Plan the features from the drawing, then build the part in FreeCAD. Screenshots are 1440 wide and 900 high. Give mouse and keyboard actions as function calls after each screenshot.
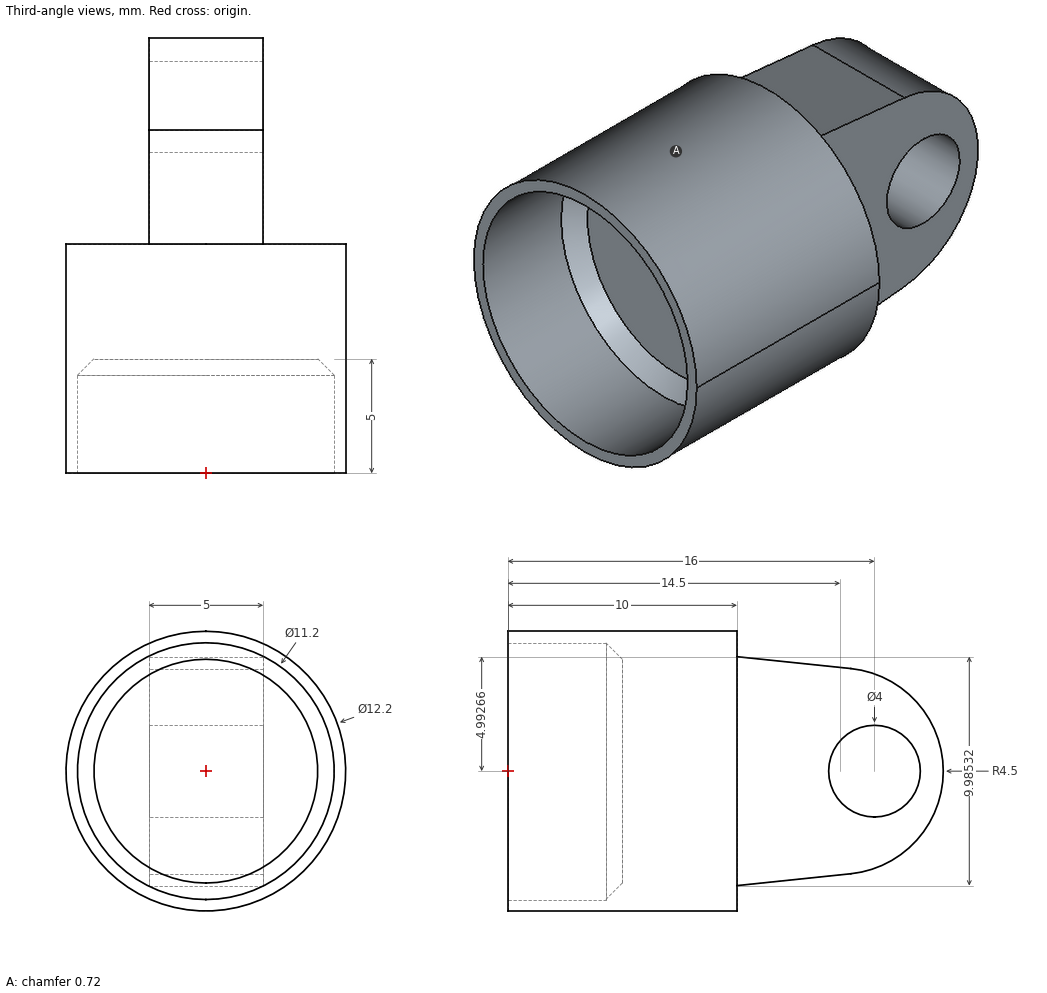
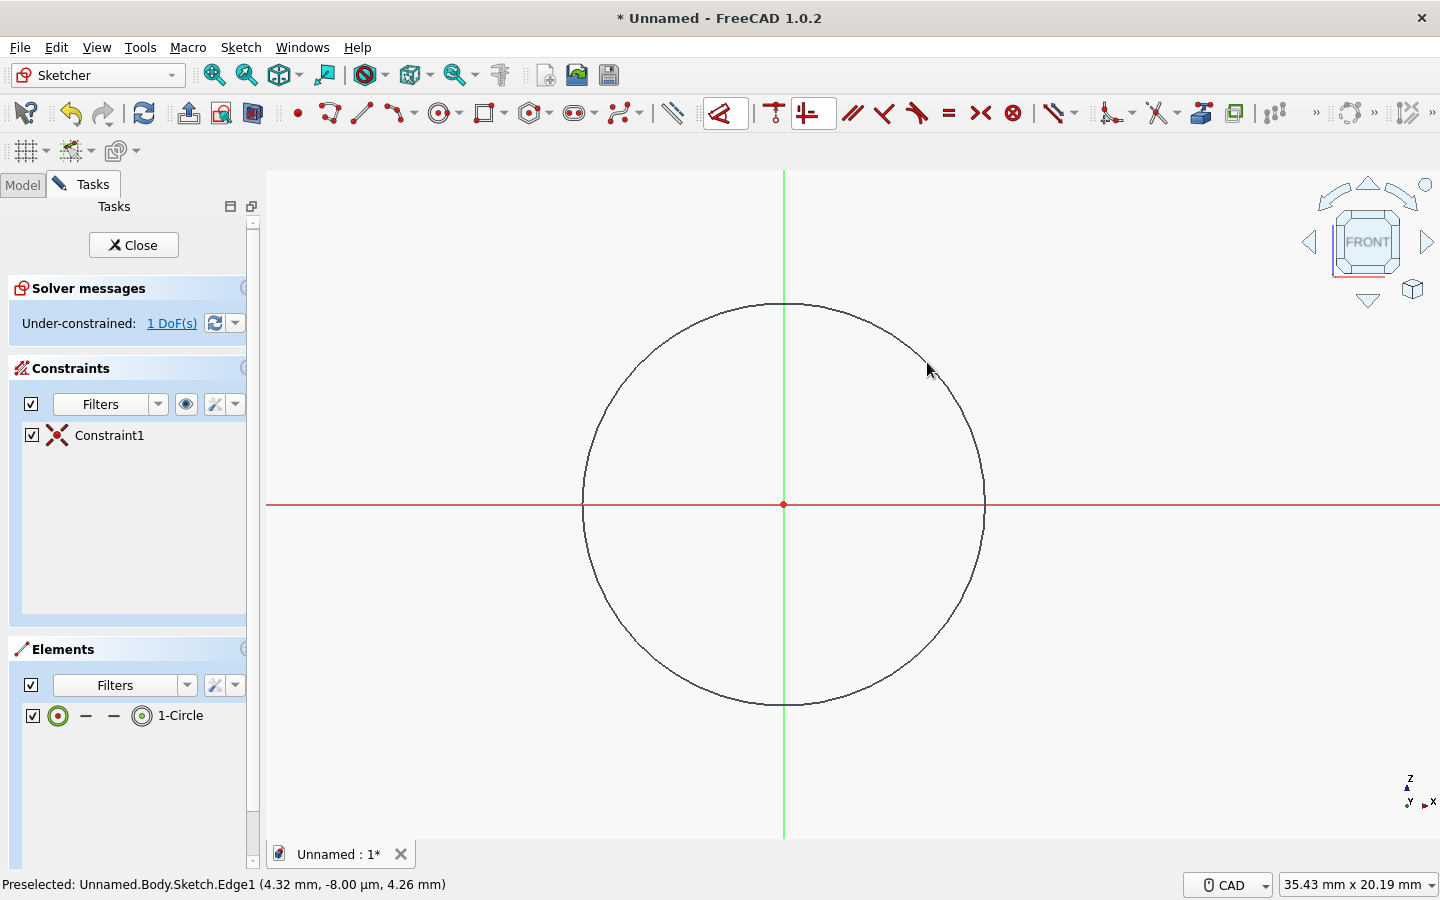
key(d)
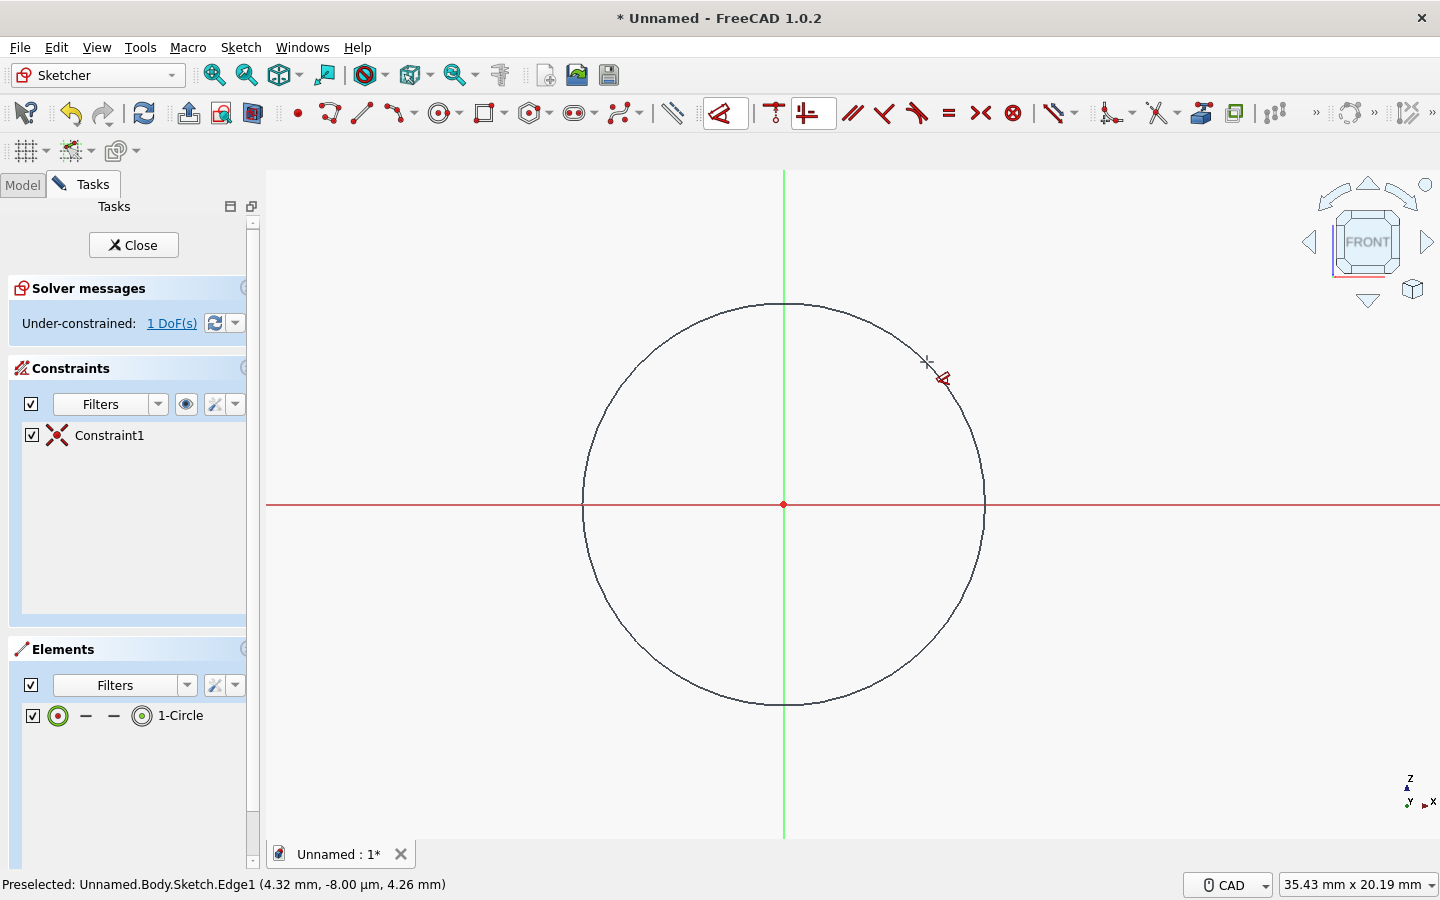
click(926, 362)
click(949, 339)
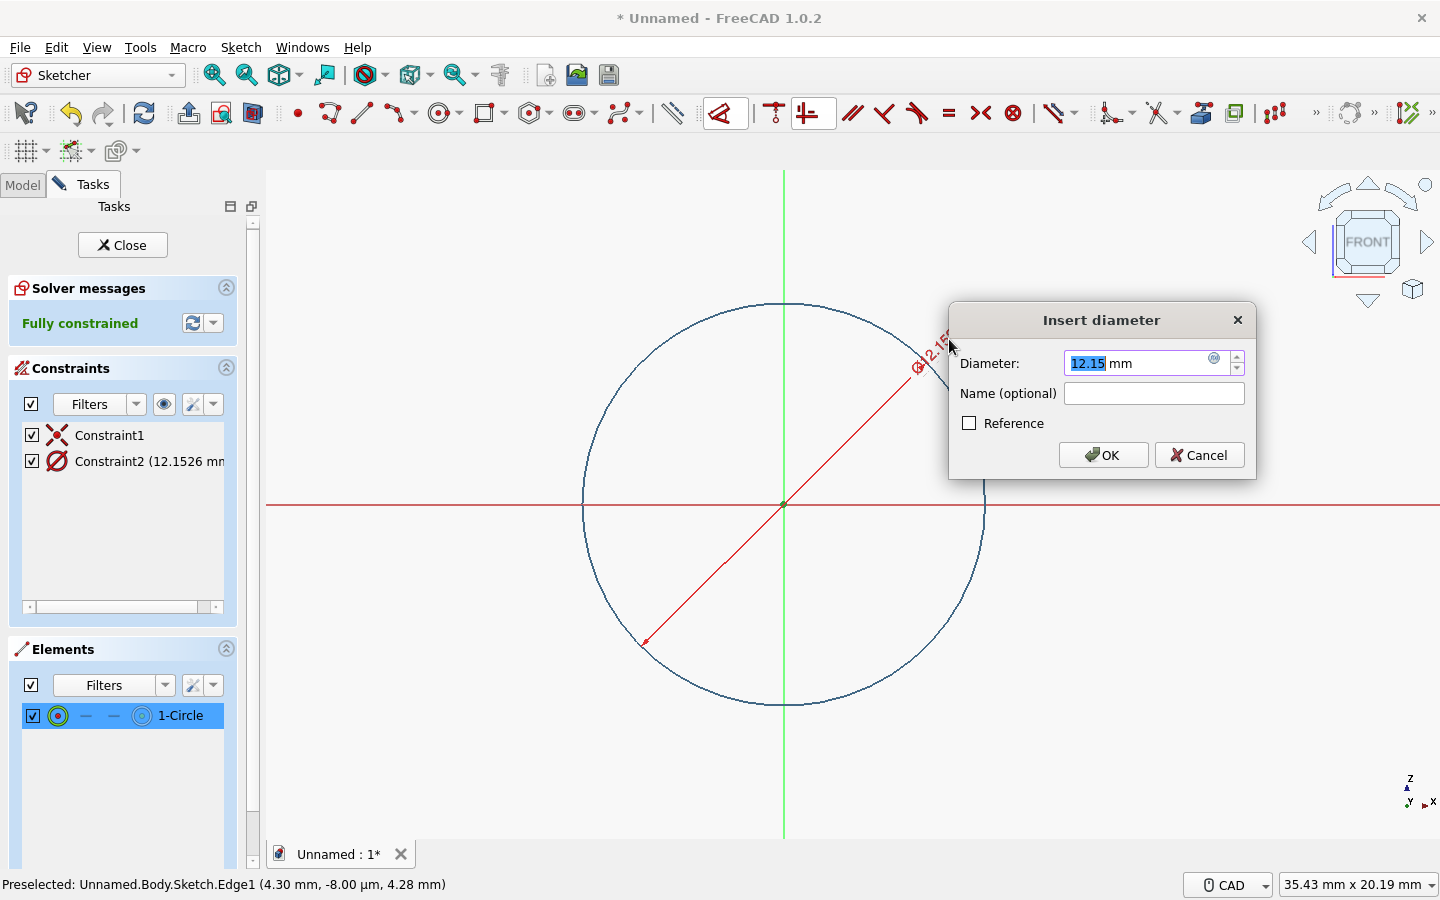
text(12.2)
key(Return)
key(Escape)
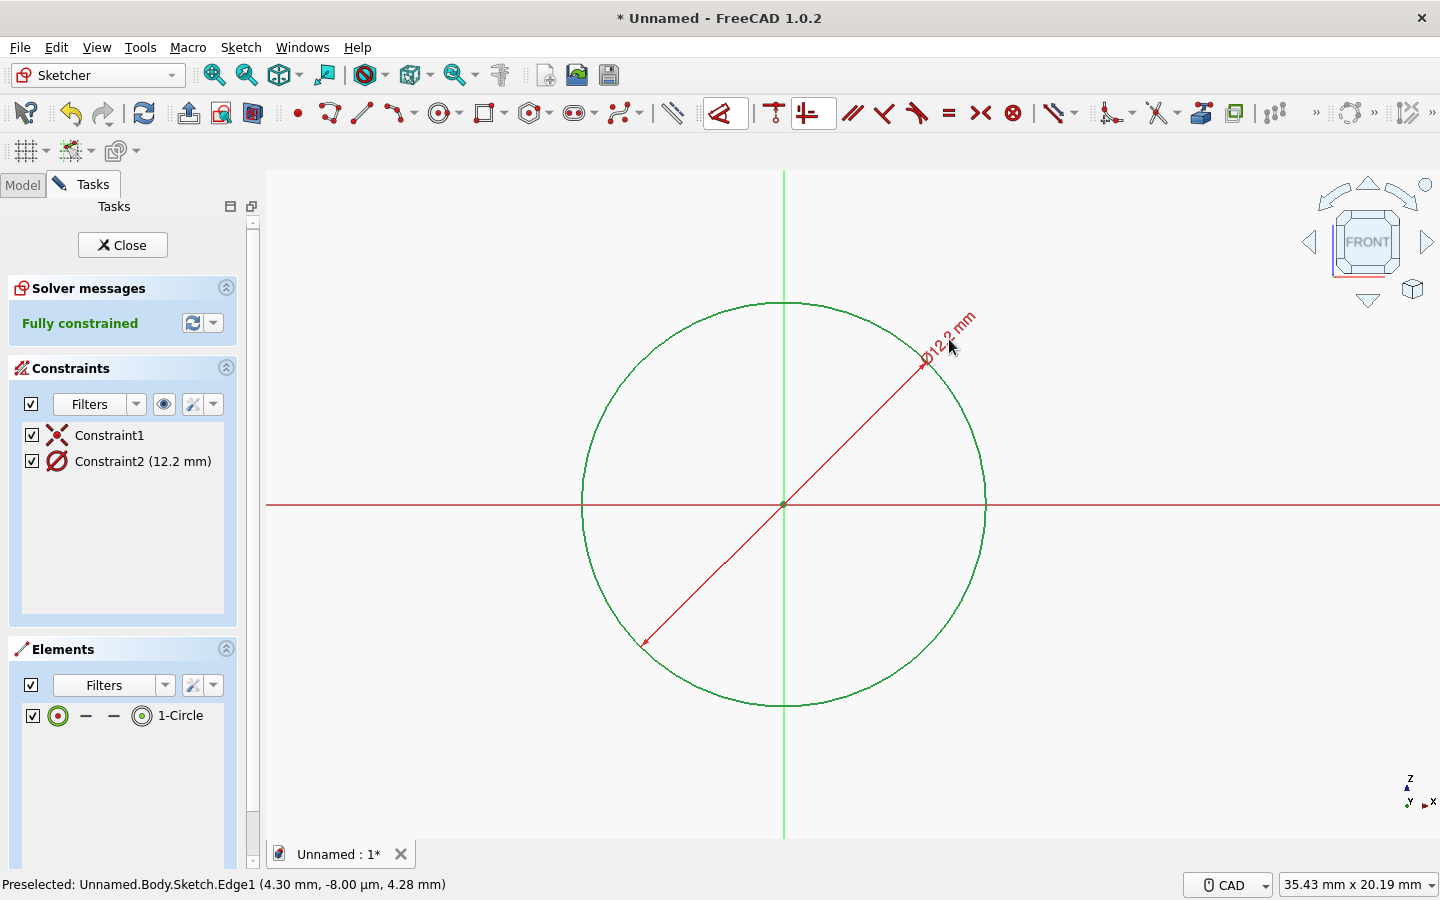
click(123, 245)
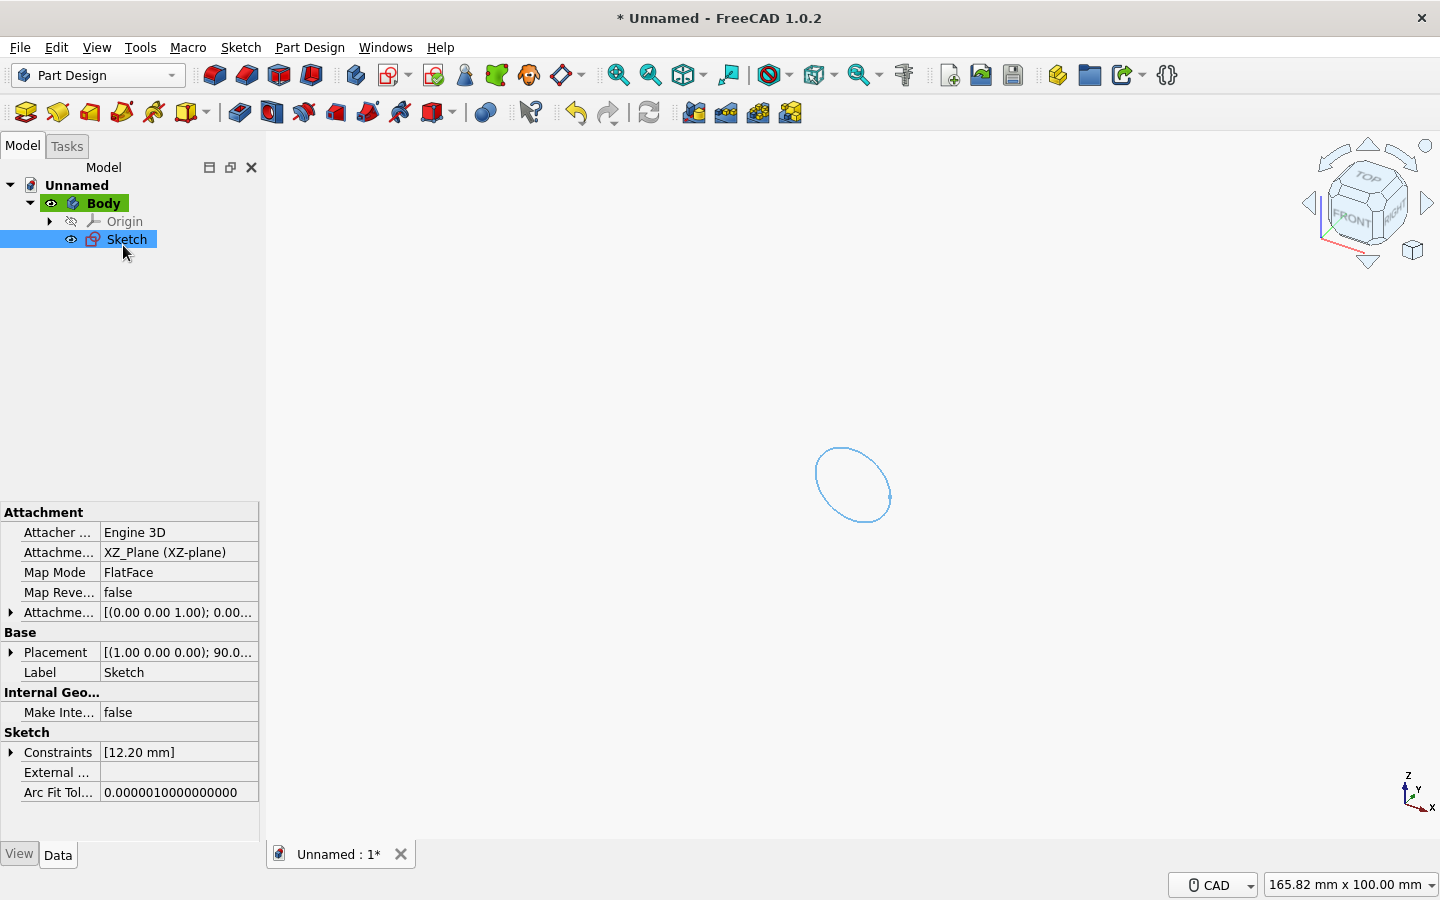
click(26, 112)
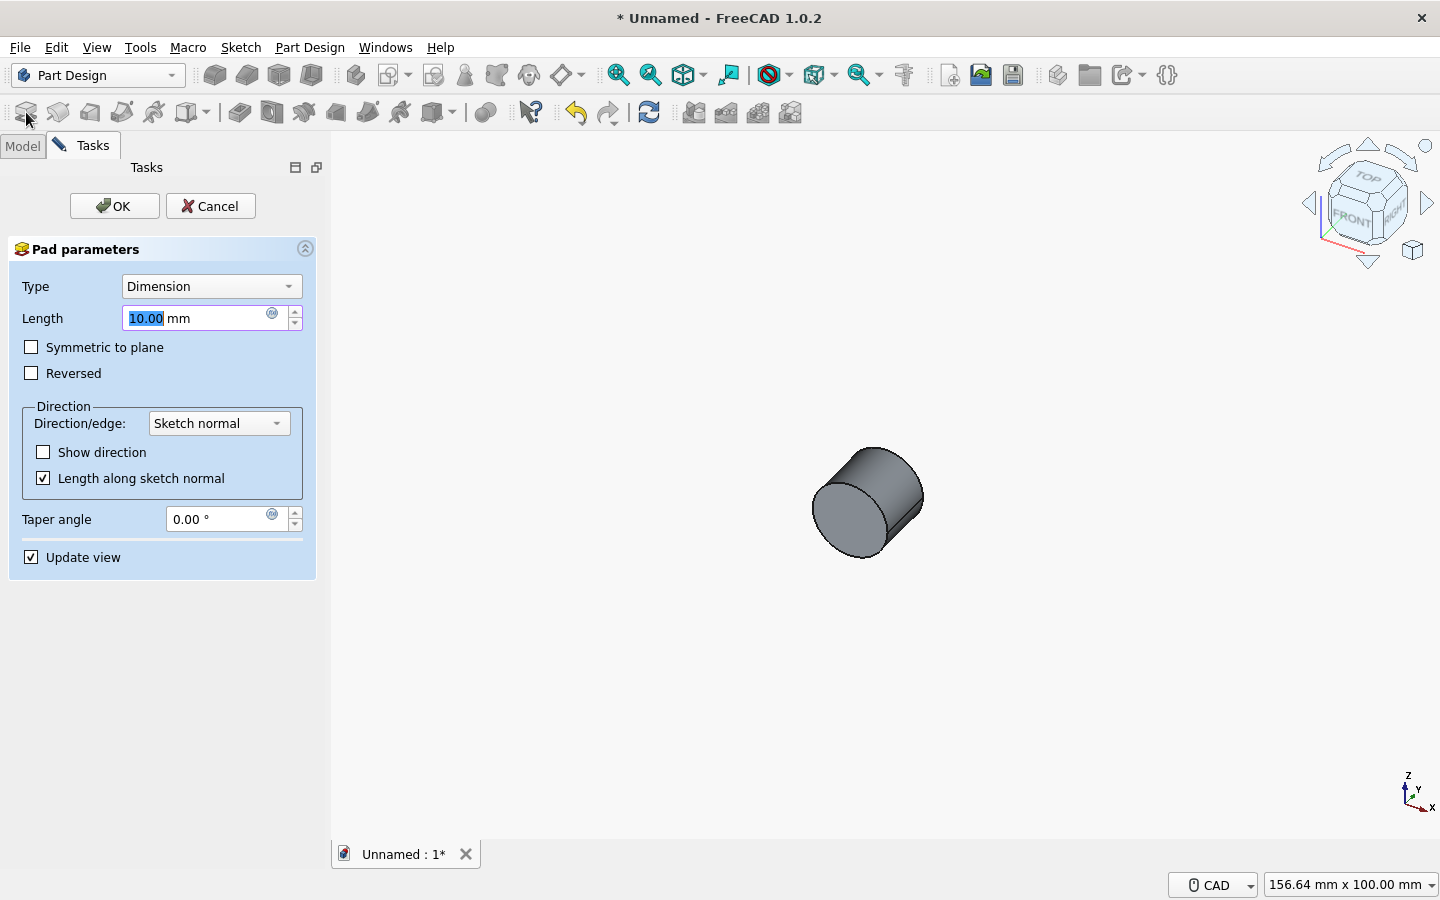
text(10)
key(Tab)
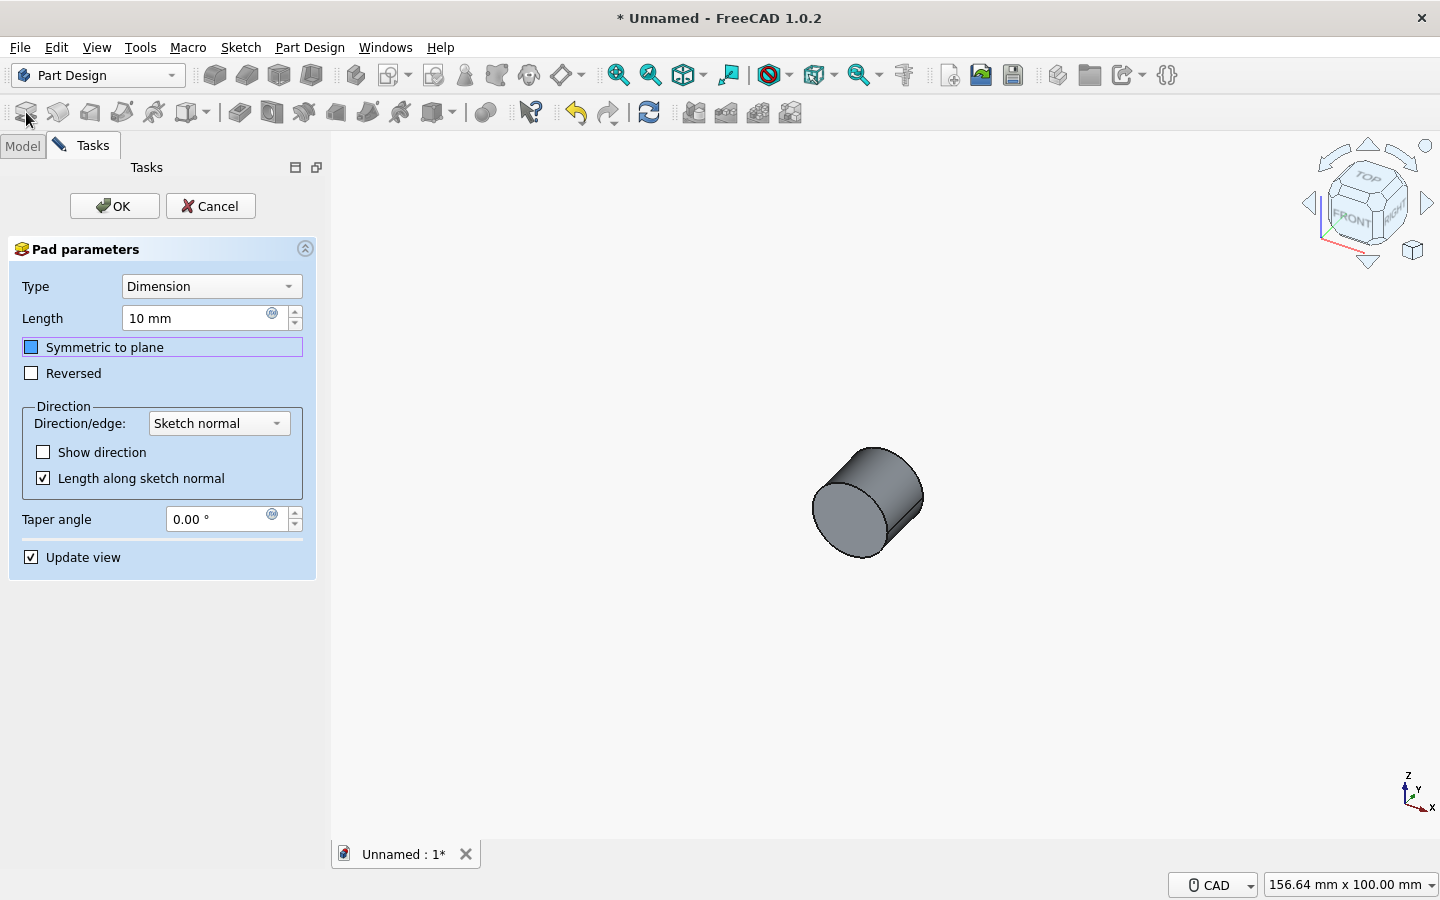
click(30, 373)